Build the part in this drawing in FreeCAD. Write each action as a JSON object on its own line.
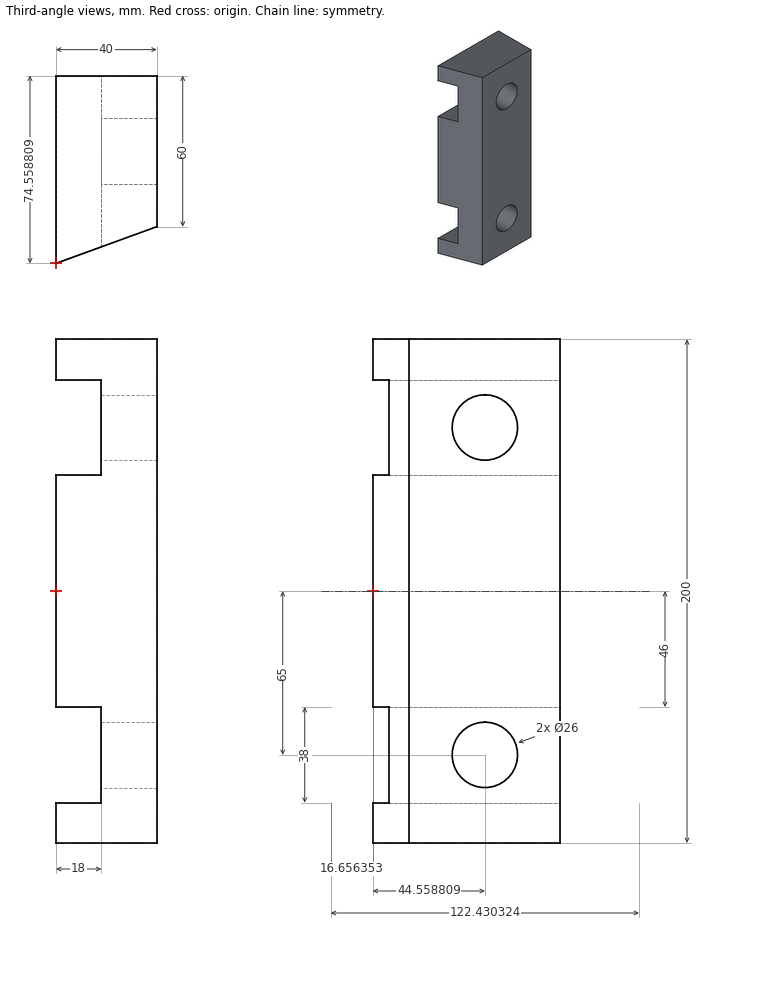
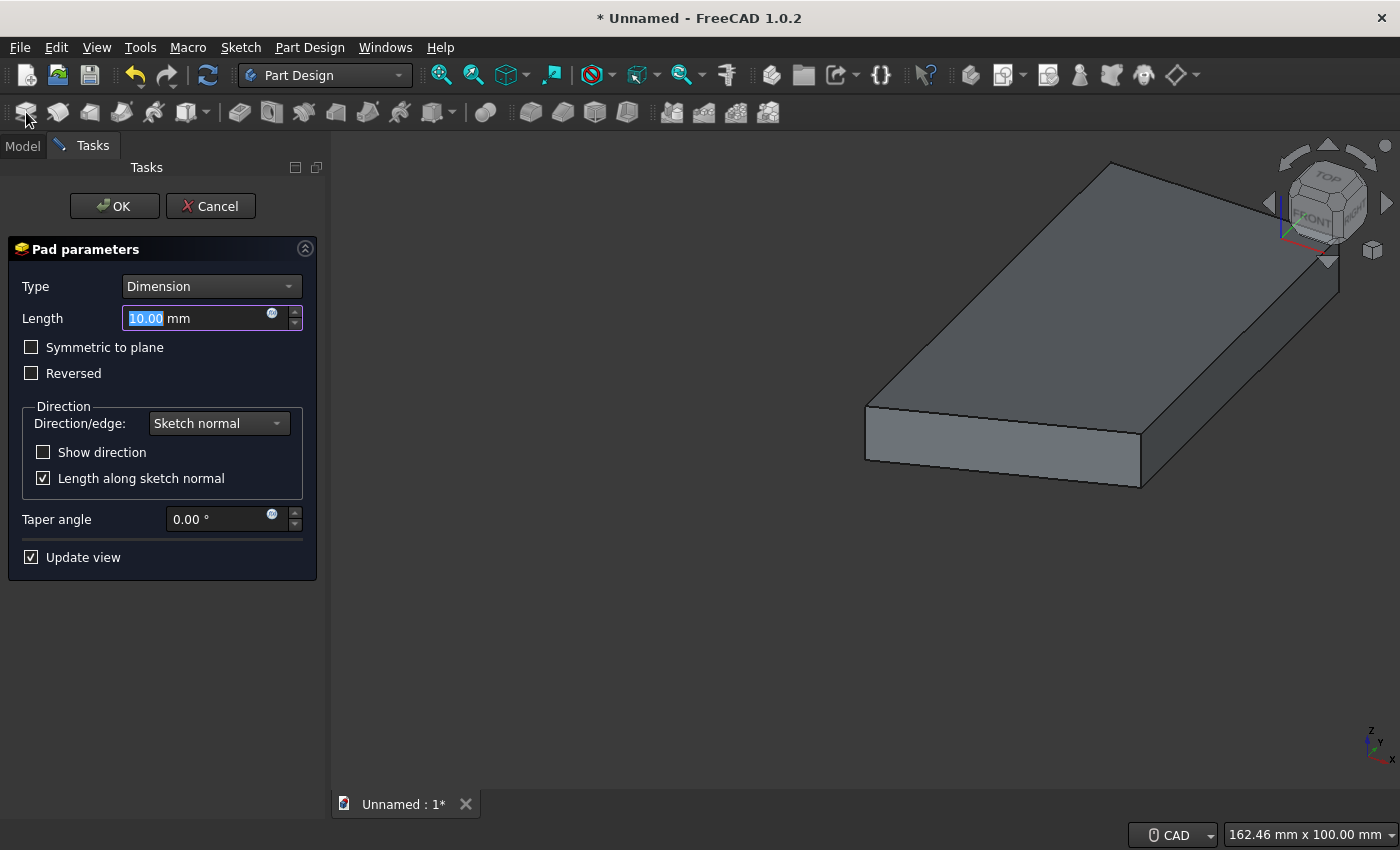
{"action": "type", "text": "200"}
{"action": "key", "text": "Tab"}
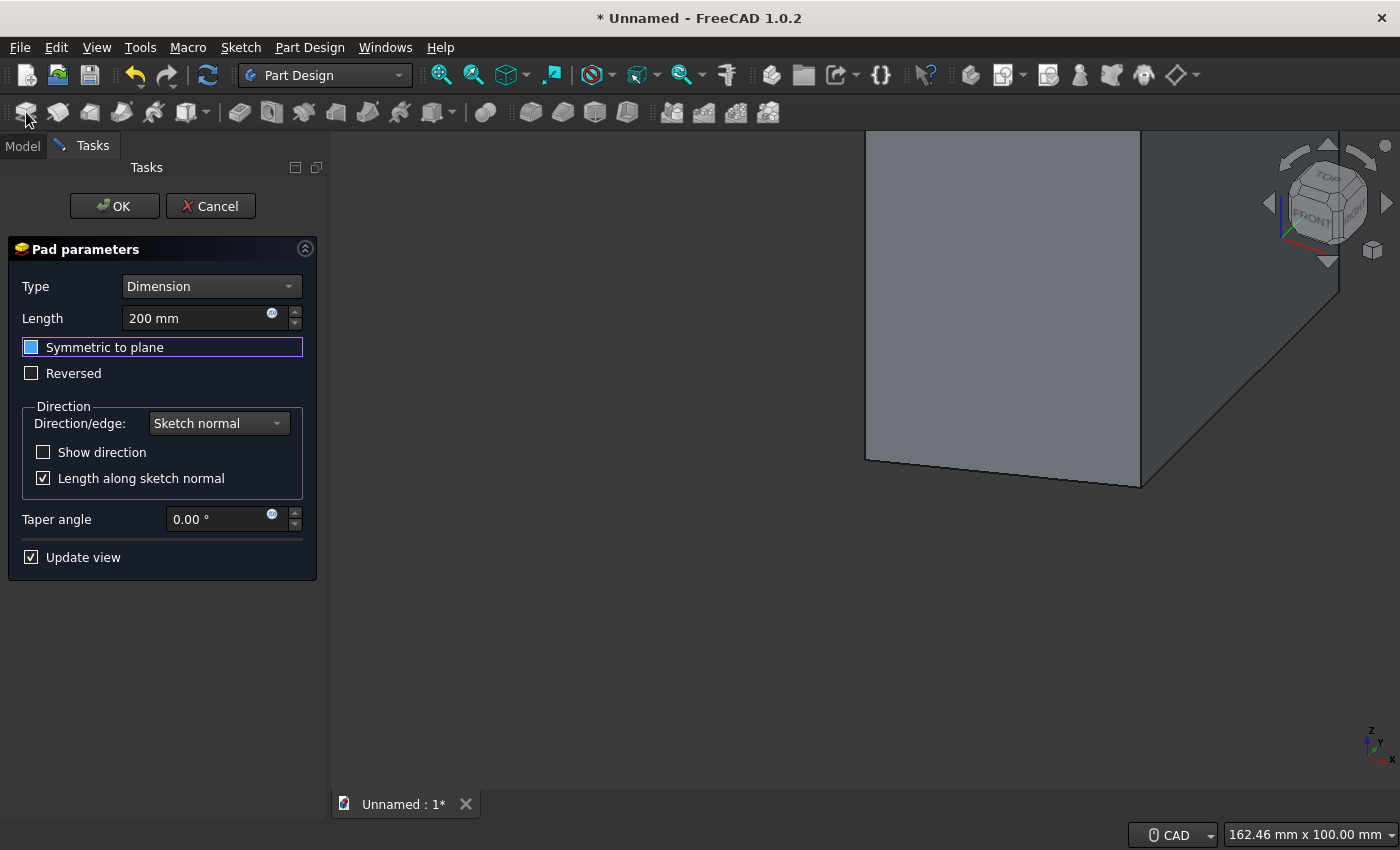
{"action": "left_click", "coordinate": [30, 347]}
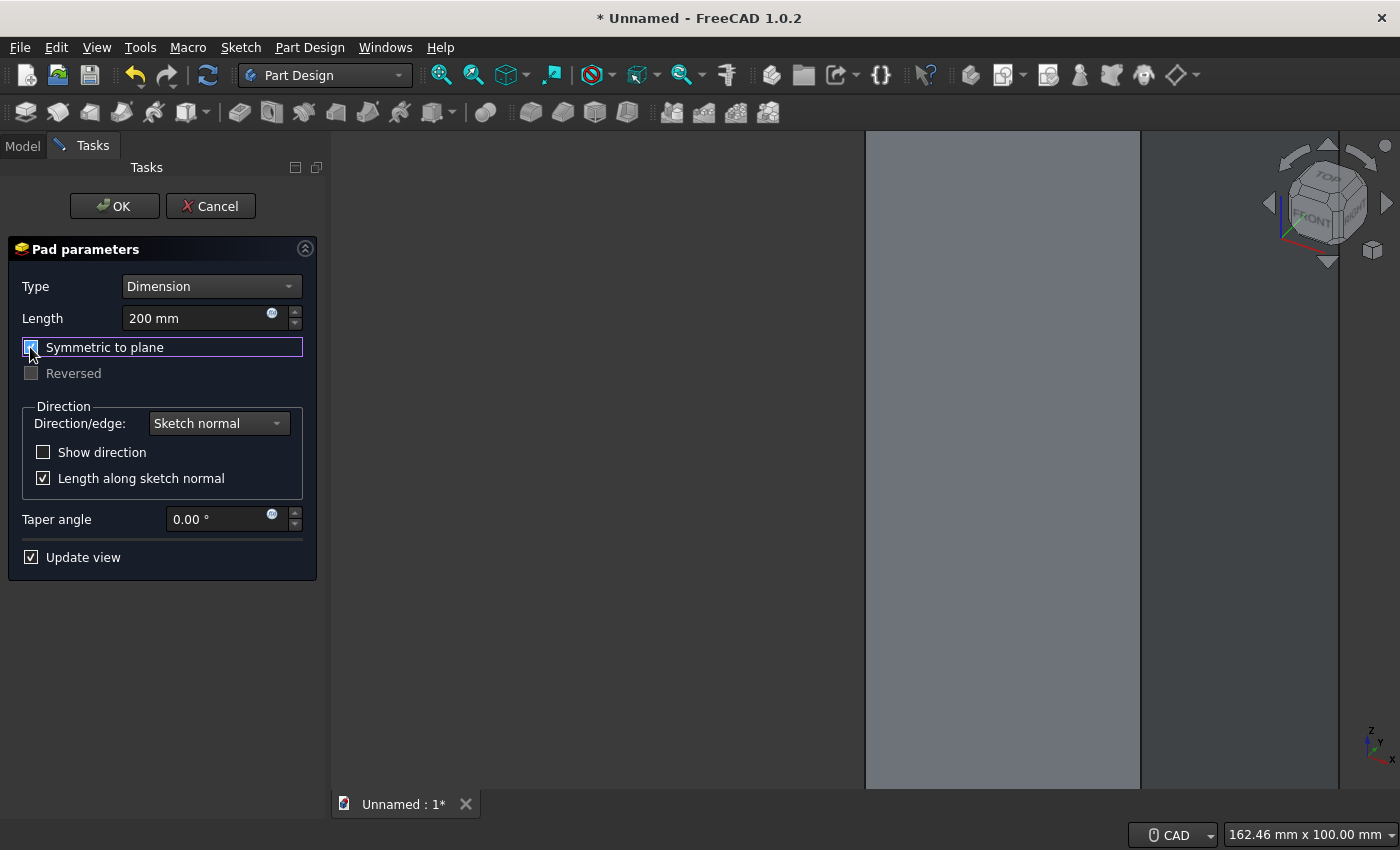
{"action": "left_click", "coordinate": [115, 206]}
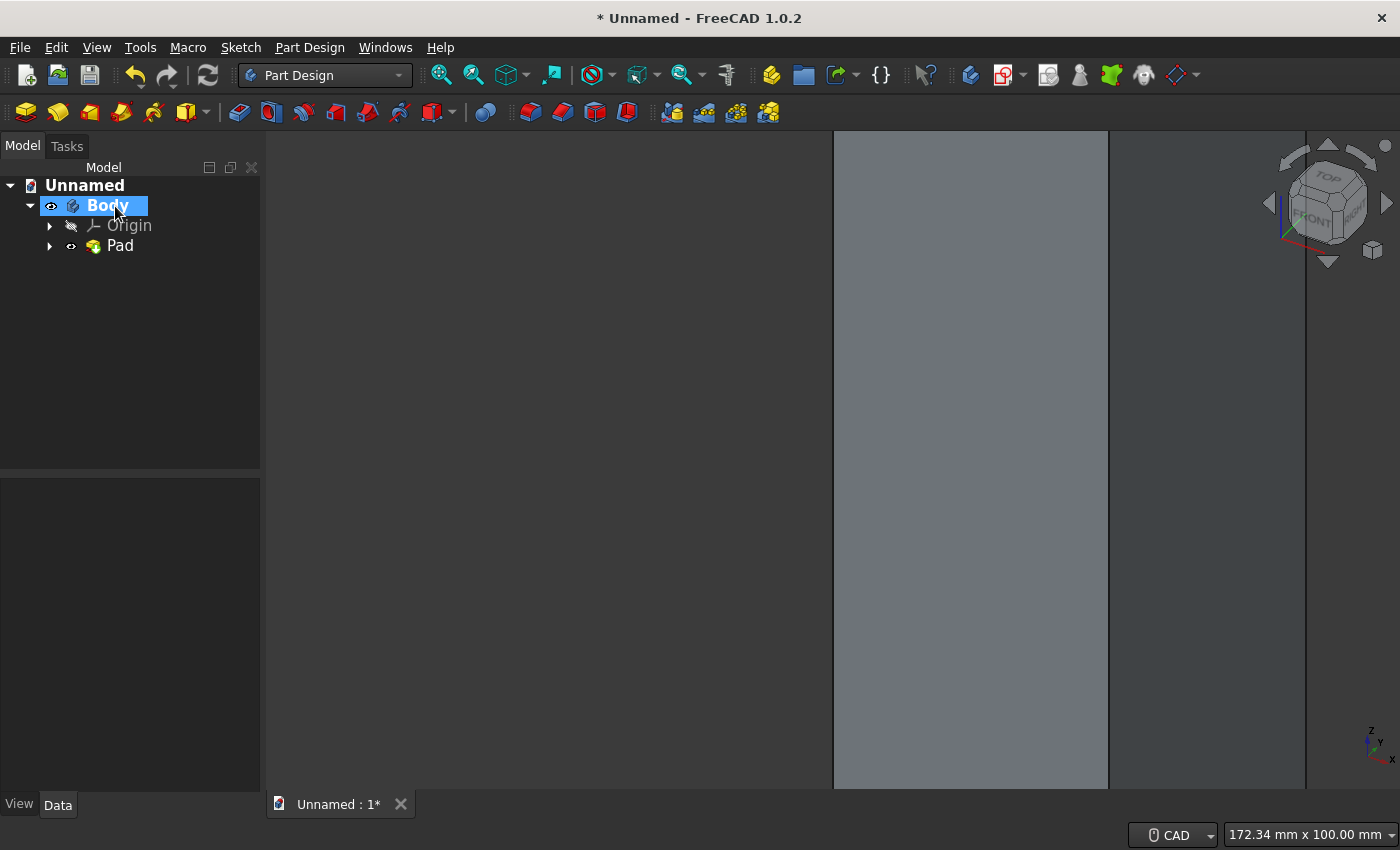
{"action": "left_click", "coordinate": [442, 76]}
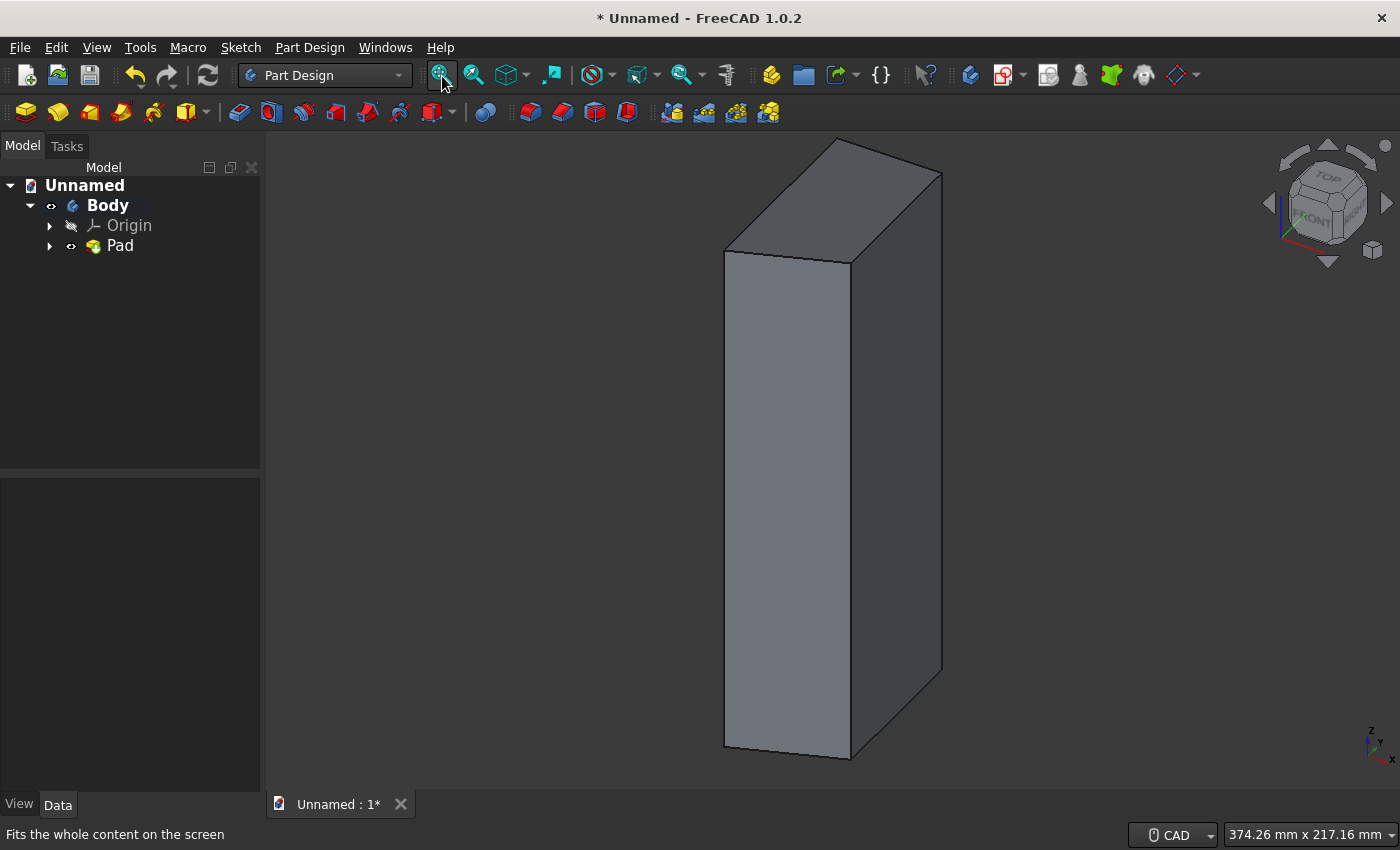
{"action": "key", "text": "6"}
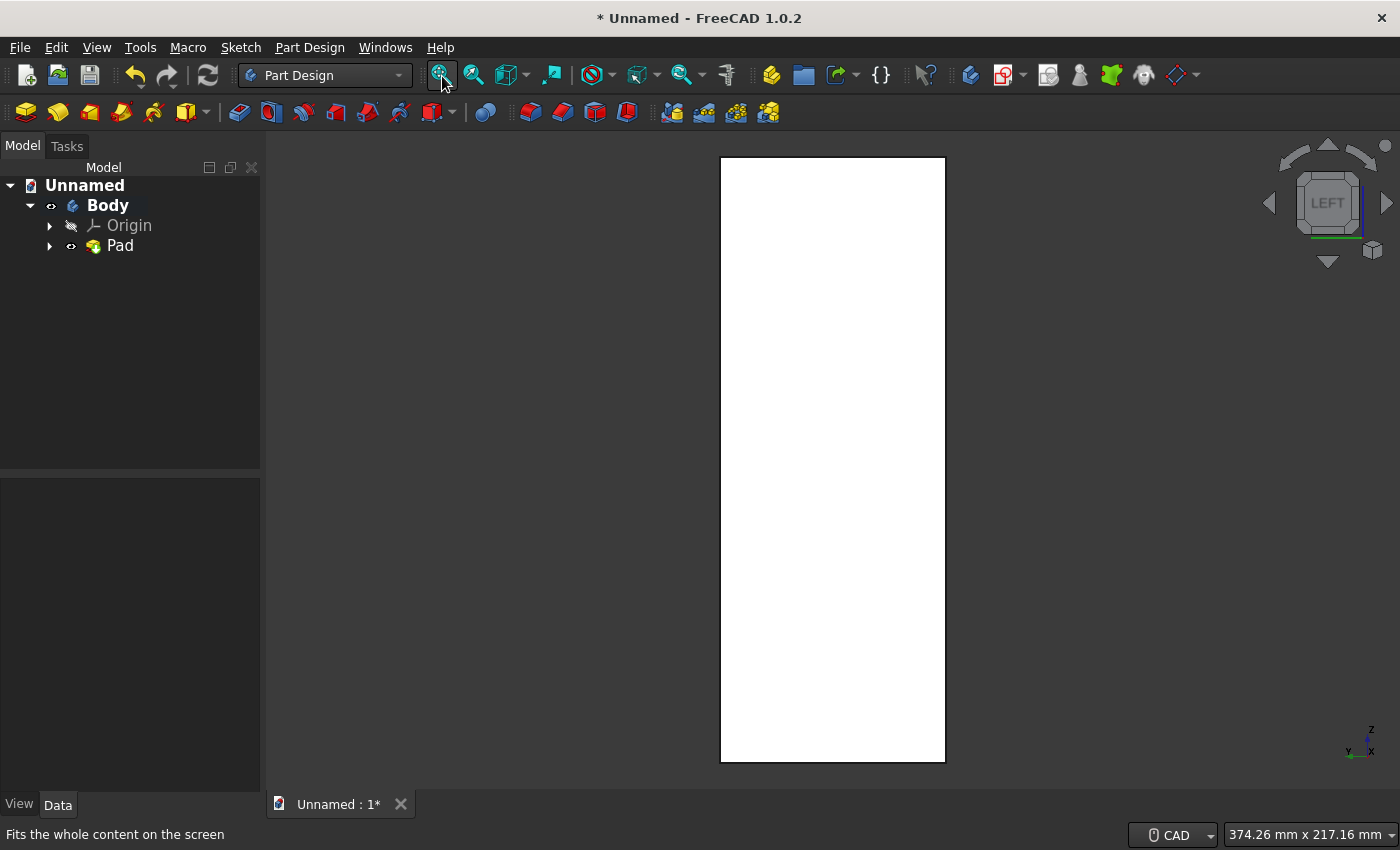
{"action": "left_click", "coordinate": [833, 286]}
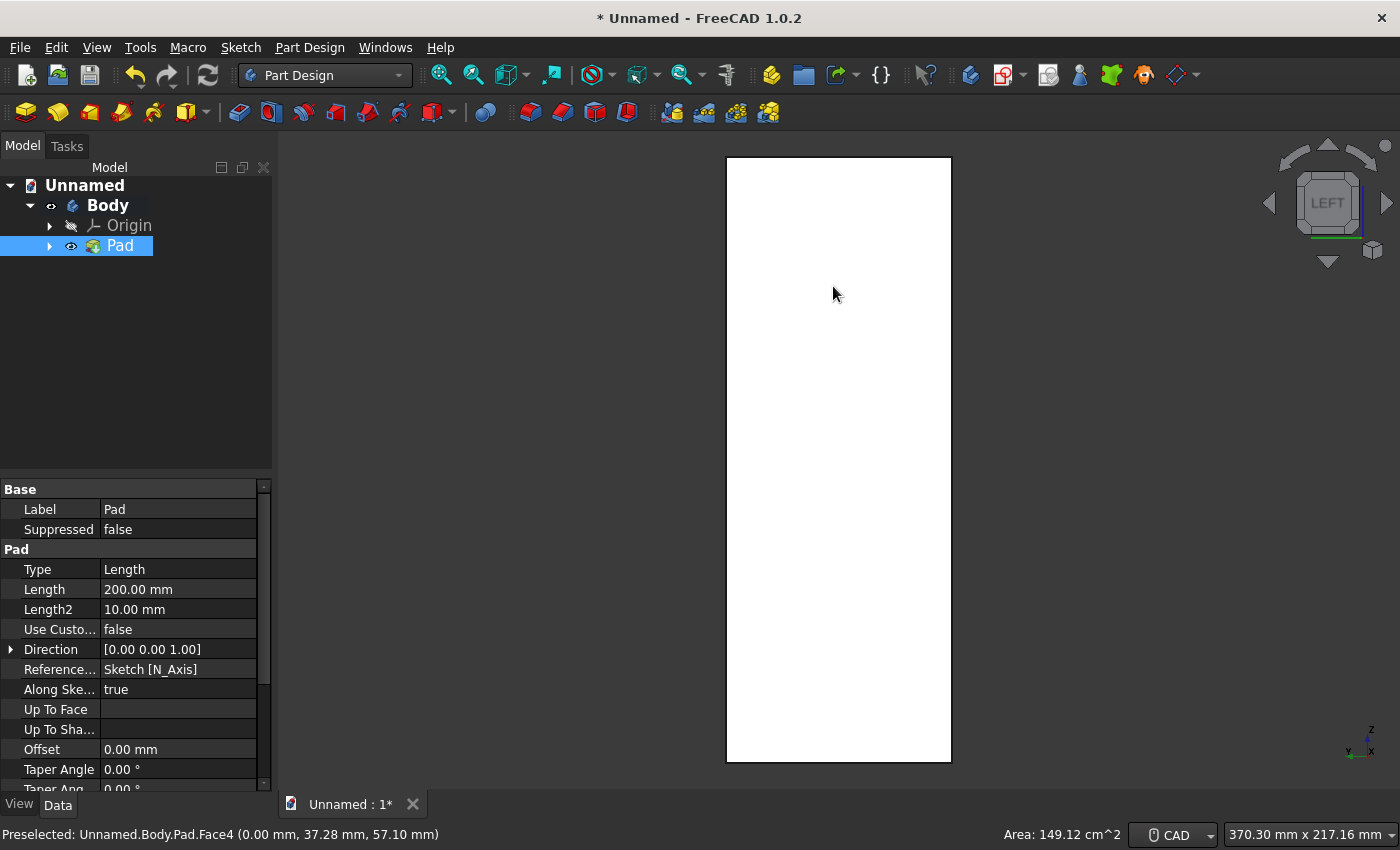
{"action": "left_click", "coordinate": [1004, 76]}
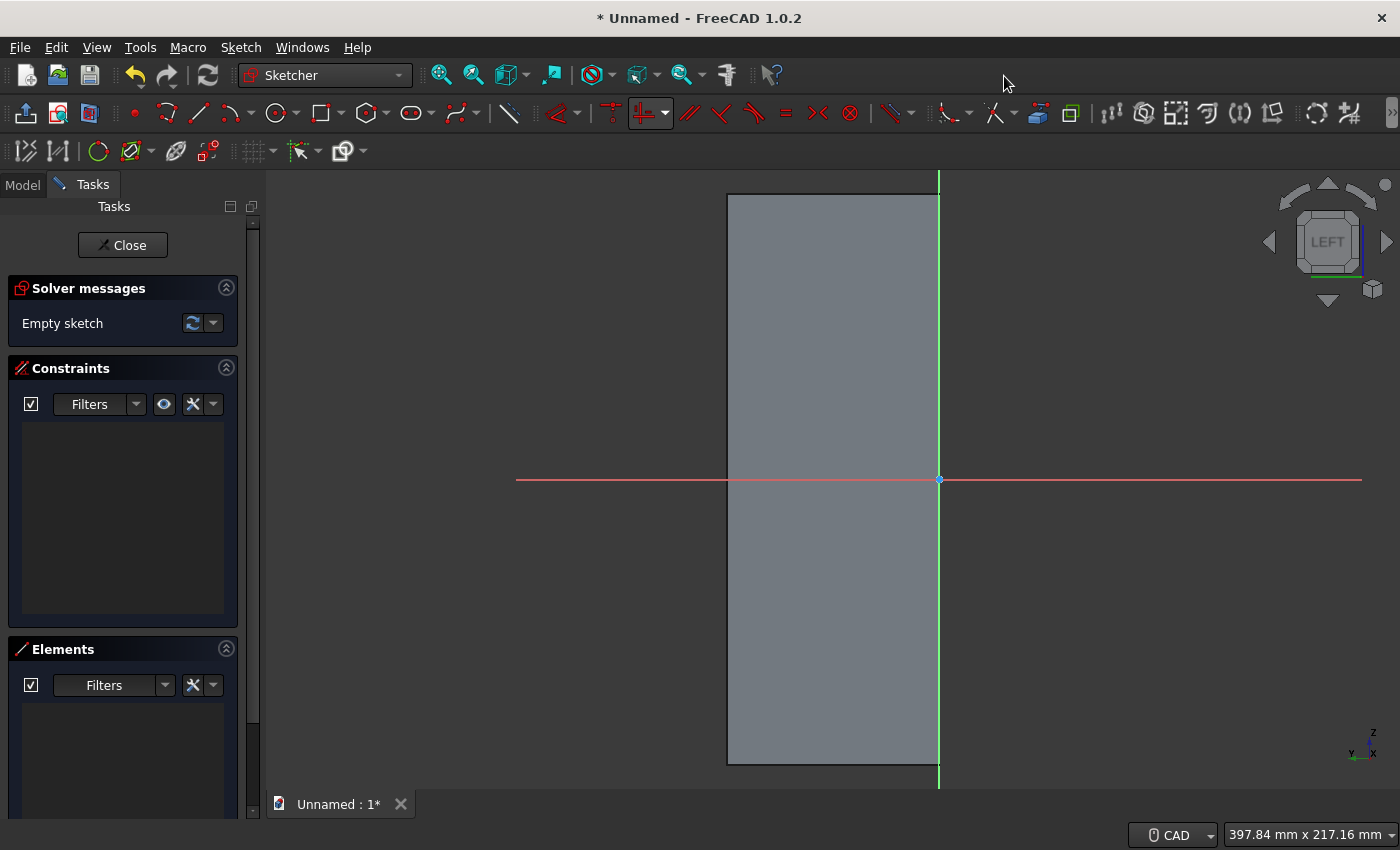
{"action": "scroll", "coordinate": [870, 745], "scroll_direction": "up", "scroll_amount": 3}